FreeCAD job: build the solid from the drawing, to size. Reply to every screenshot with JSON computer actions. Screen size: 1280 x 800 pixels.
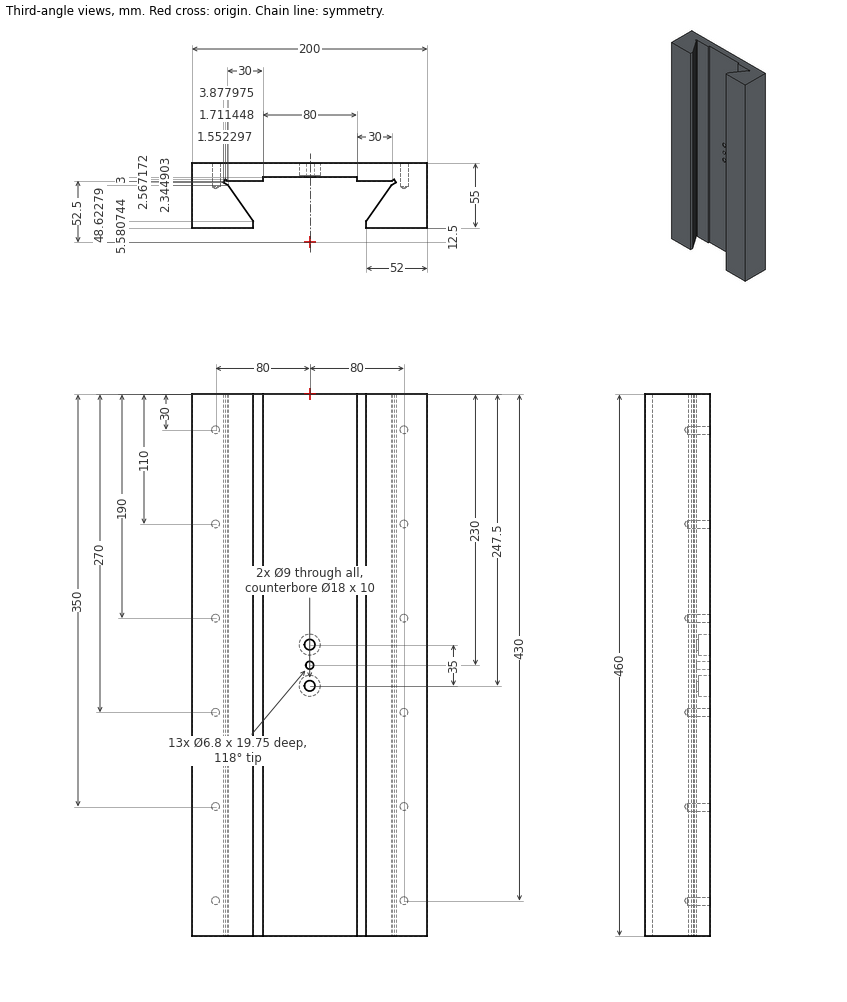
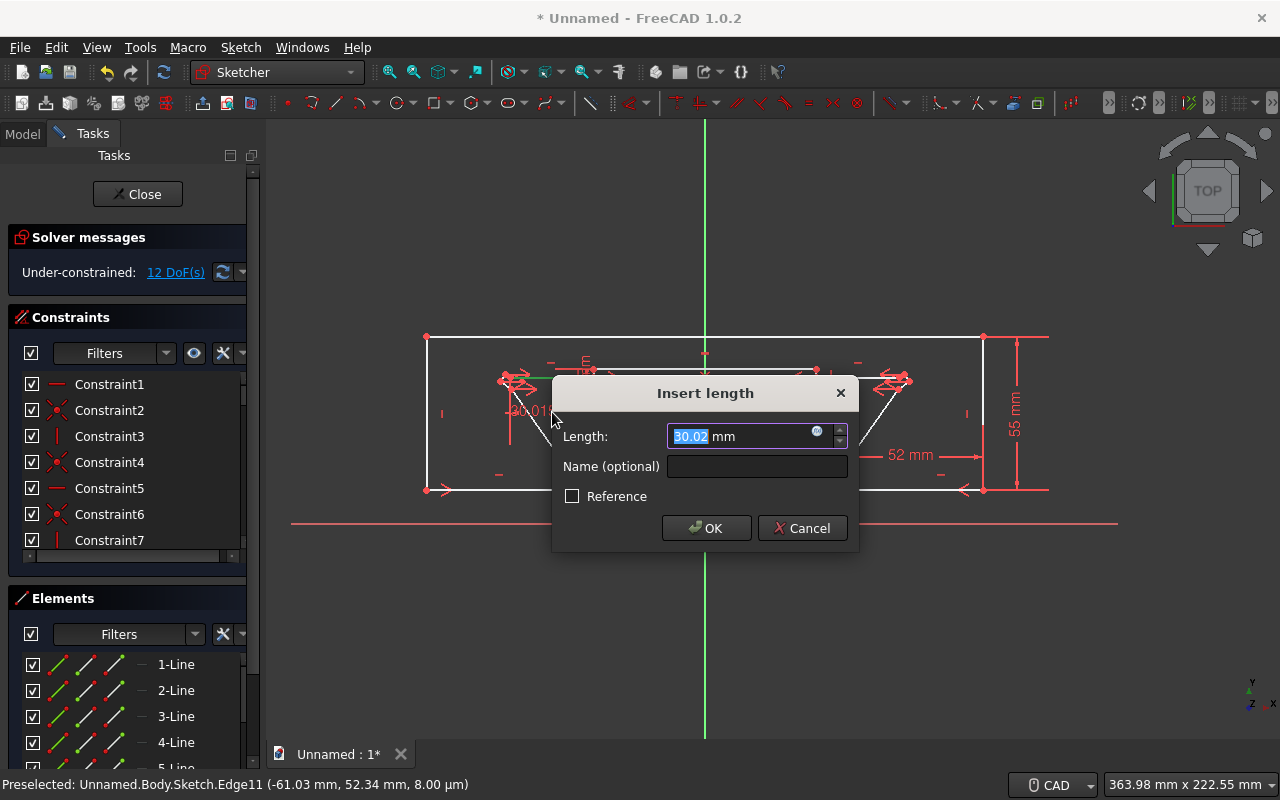
{"action": "type", "text": "30"}
{"action": "key", "text": "Return"}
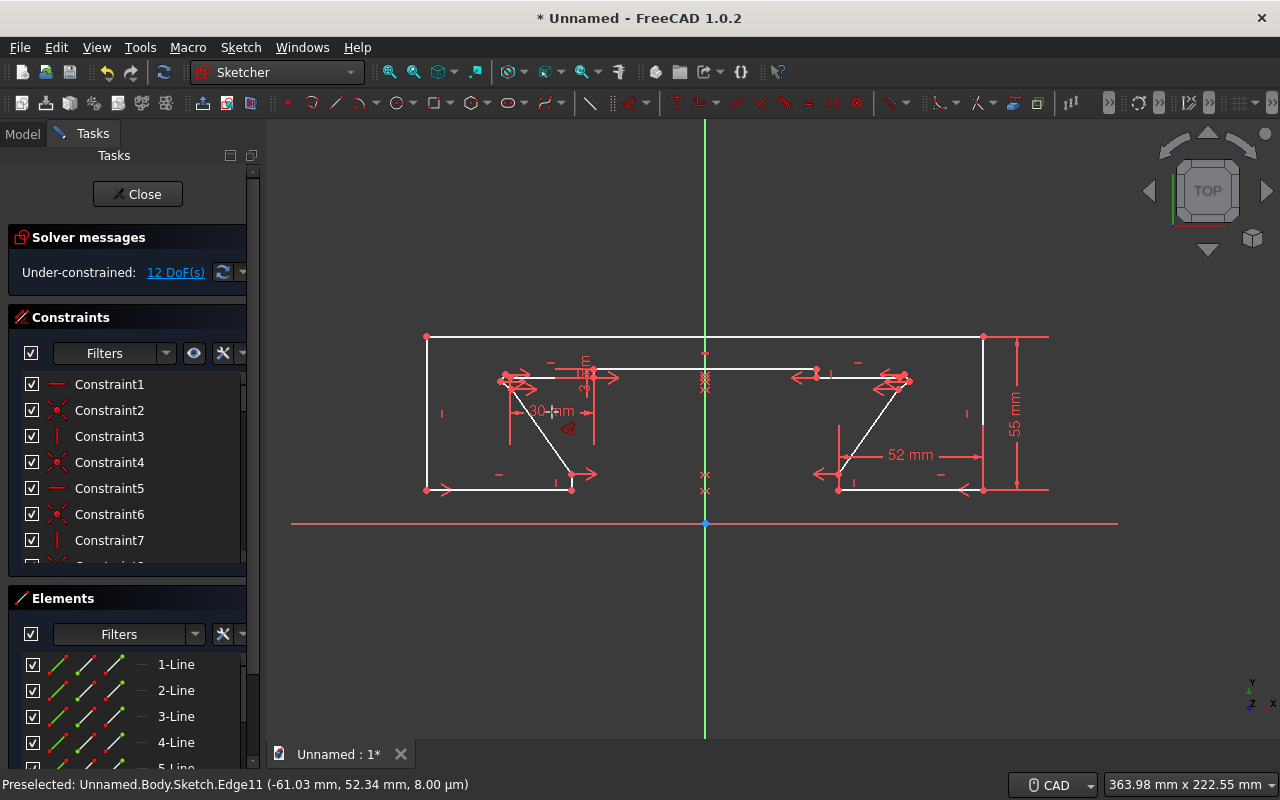
{"action": "left_click", "coordinate": [661, 369]}
{"action": "left_click", "coordinate": [654, 403]}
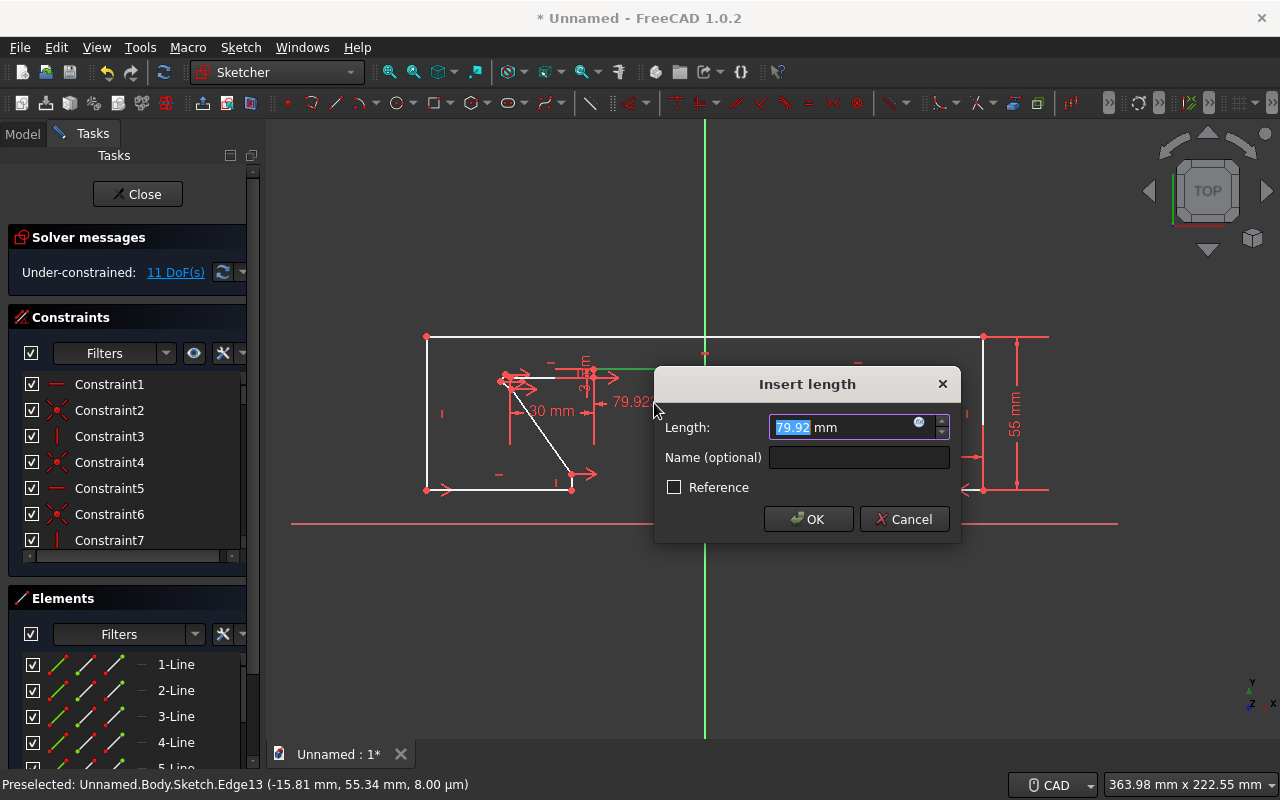
{"action": "type", "text": "80"}
{"action": "key", "text": "Return"}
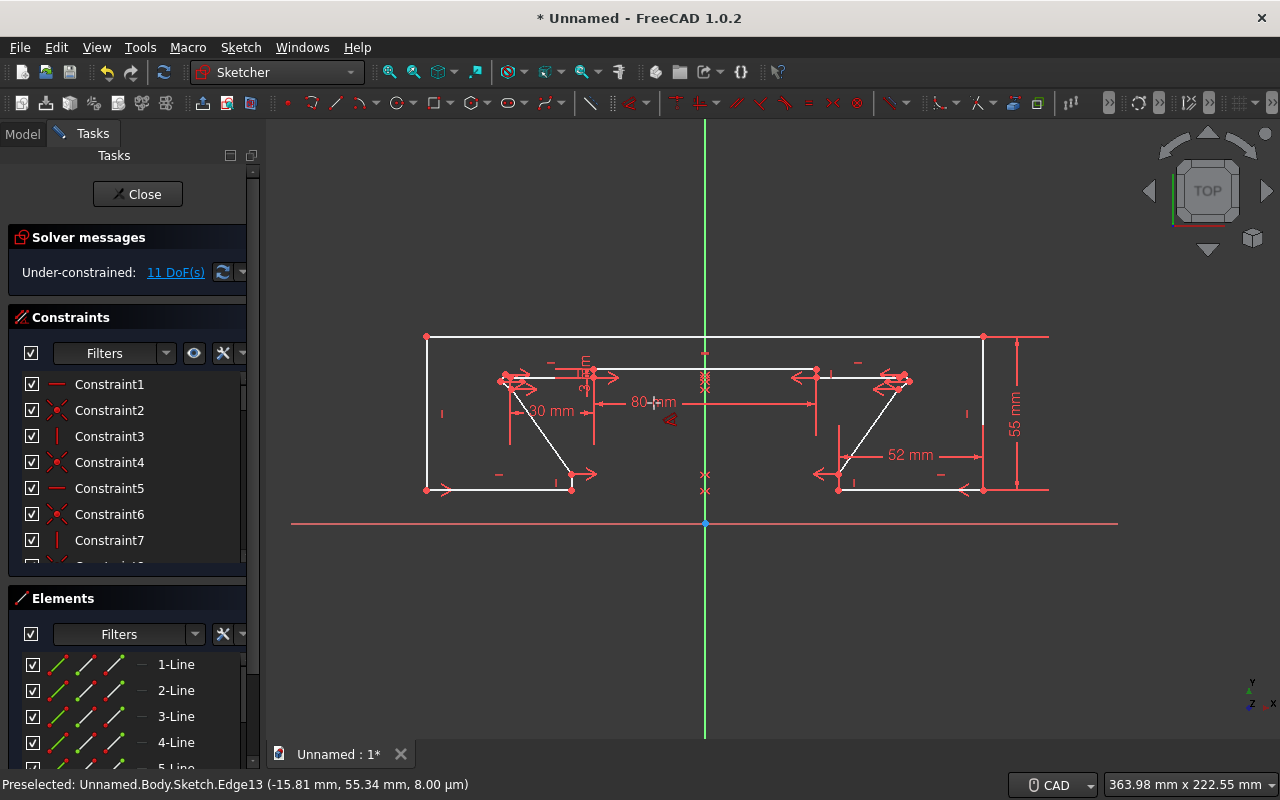
{"action": "left_click", "coordinate": [842, 378]}
{"action": "left_click", "coordinate": [858, 412]}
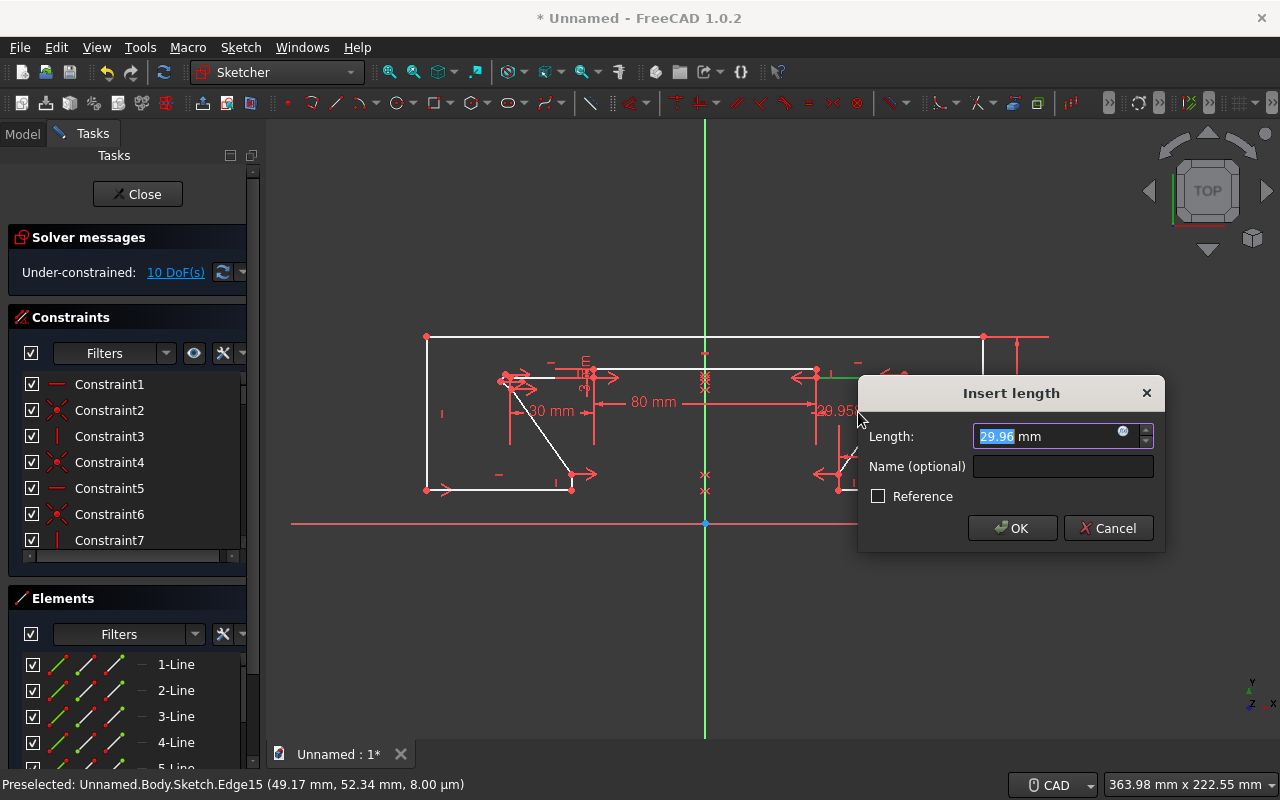
{"action": "type", "text": "30"}
{"action": "key", "text": "Return"}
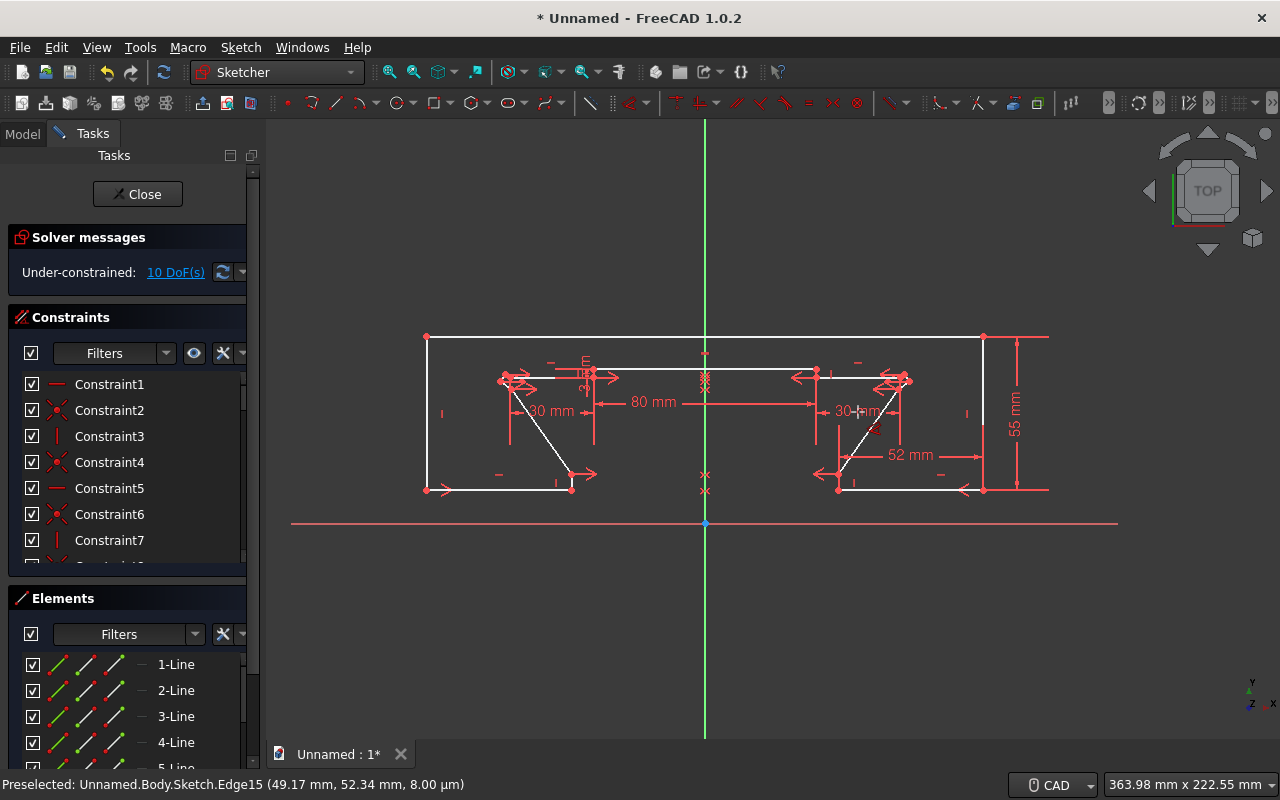
{"action": "left_click", "coordinate": [816, 337]}
{"action": "left_click", "coordinate": [577, 303]}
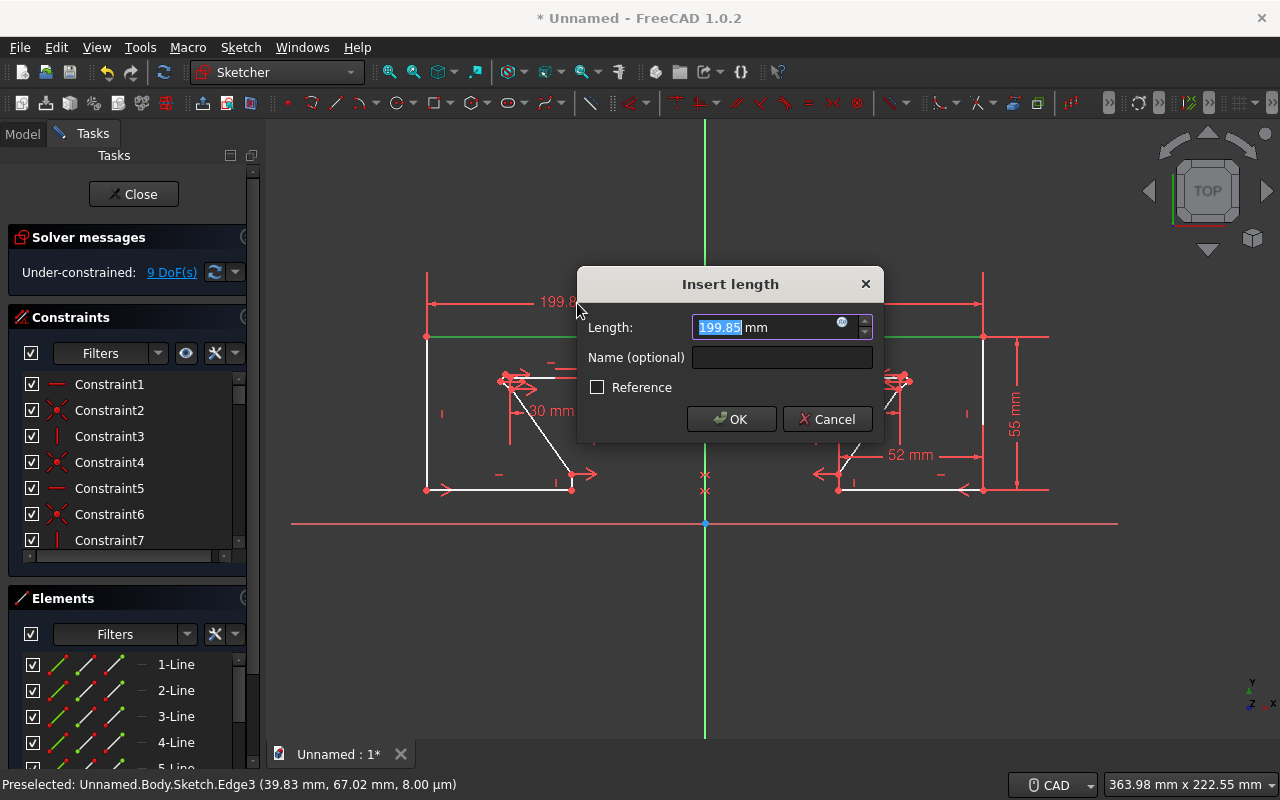
{"action": "type", "text": "200"}
{"action": "key", "text": "Return"}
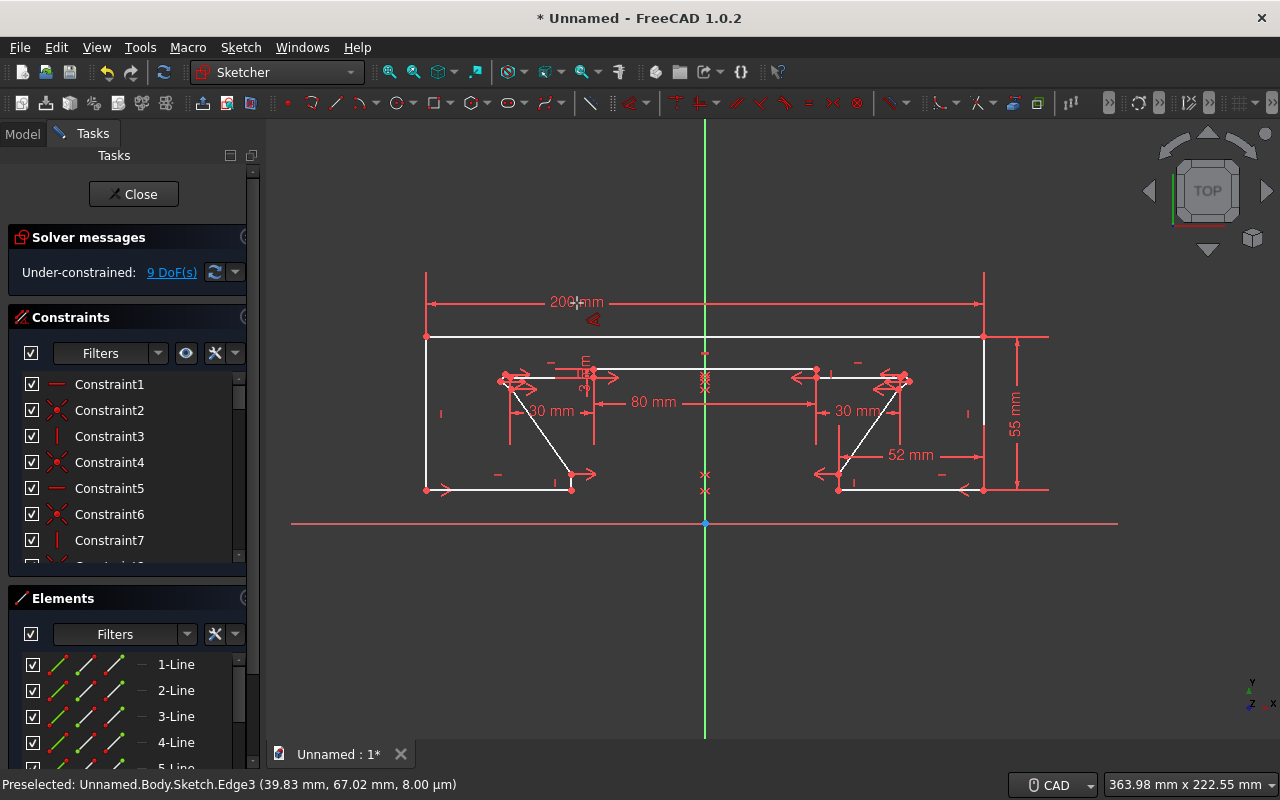
{"action": "left_click", "coordinate": [839, 490]}
{"action": "left_click", "coordinate": [873, 507]}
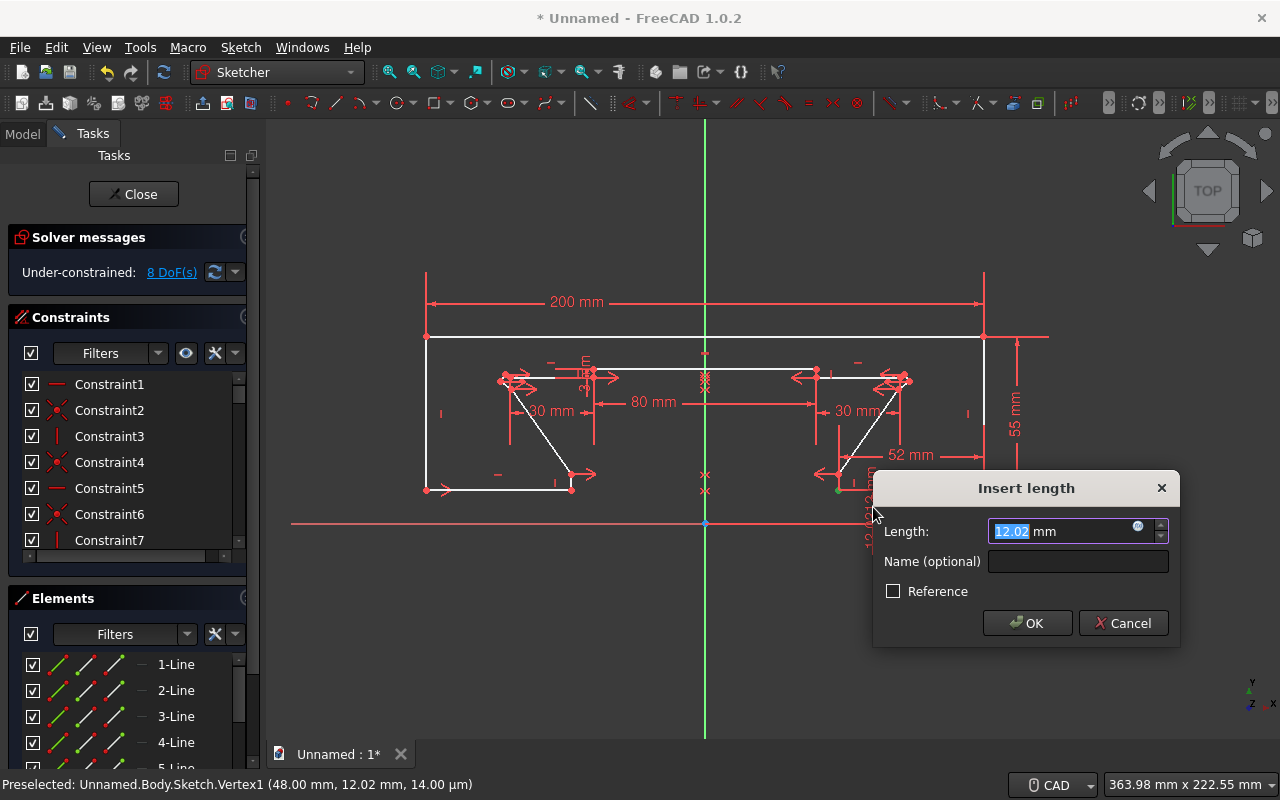
{"action": "type", "text": "12.5"}
{"action": "key", "text": "Return"}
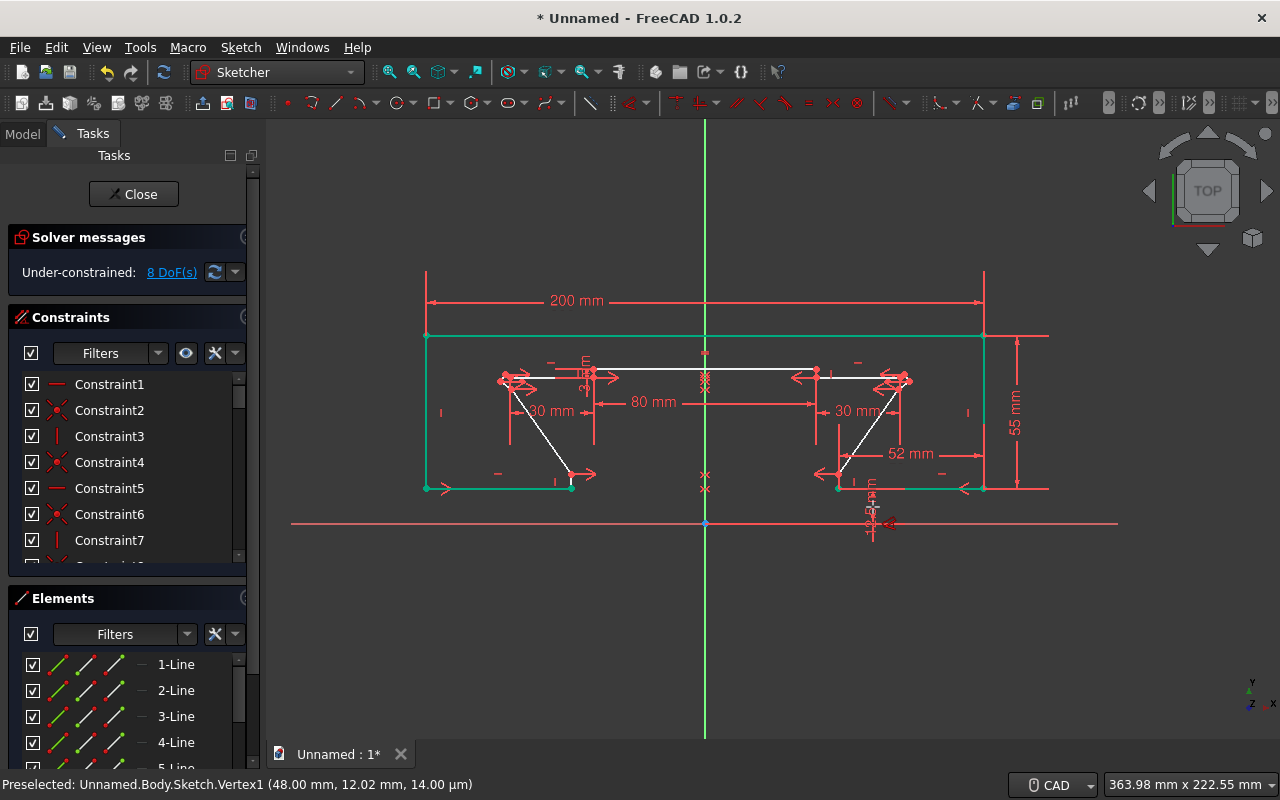
{"action": "scroll", "coordinate": [510, 378], "scroll_direction": "up", "scroll_amount": 4}